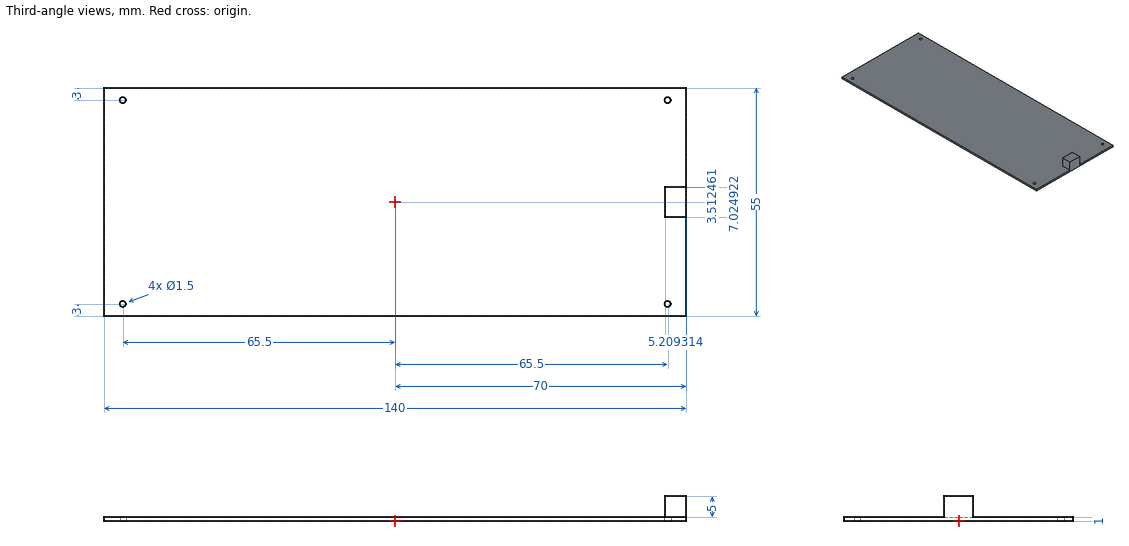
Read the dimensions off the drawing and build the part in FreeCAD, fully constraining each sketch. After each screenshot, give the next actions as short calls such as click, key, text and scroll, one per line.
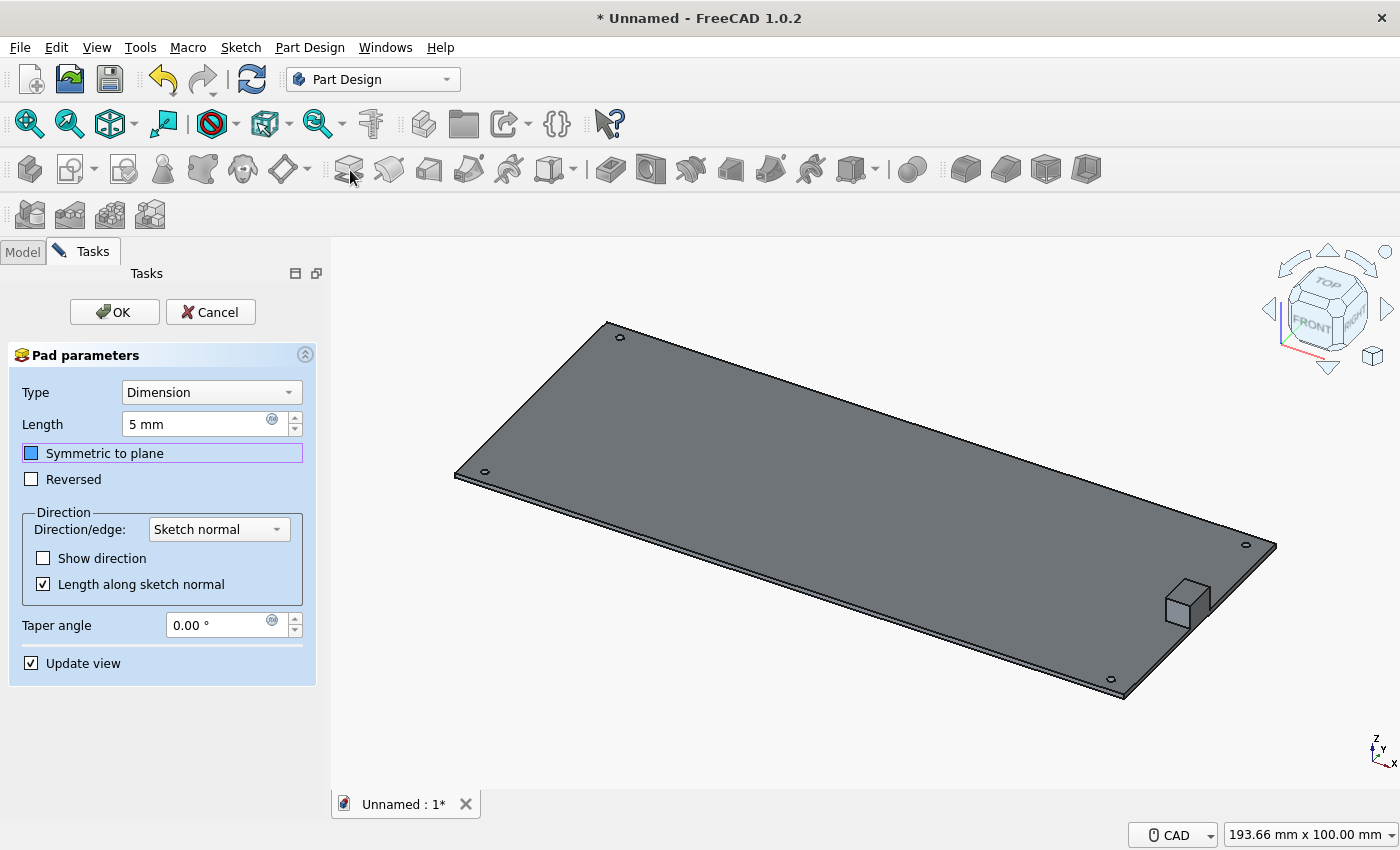
click(115, 312)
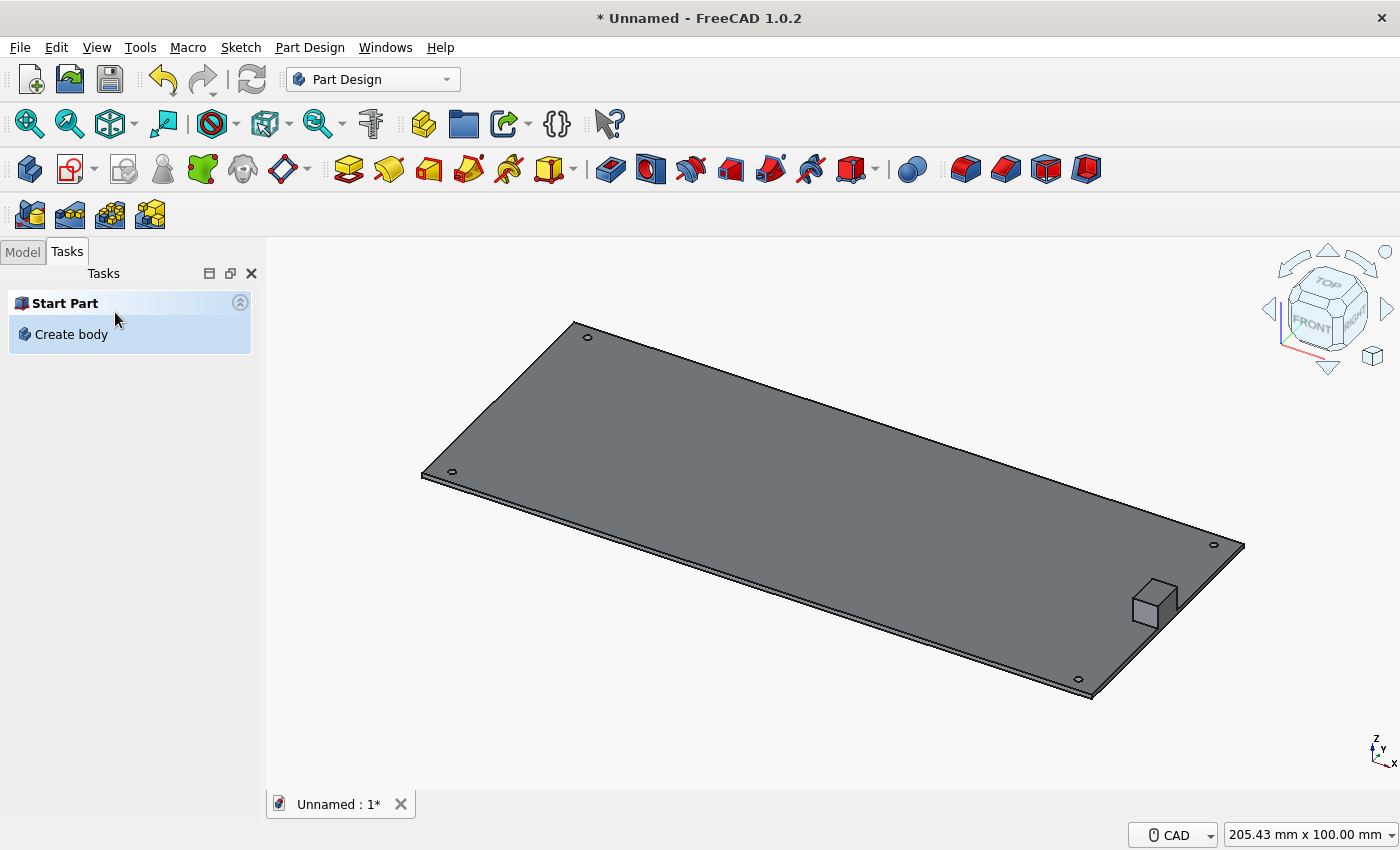
key(0)